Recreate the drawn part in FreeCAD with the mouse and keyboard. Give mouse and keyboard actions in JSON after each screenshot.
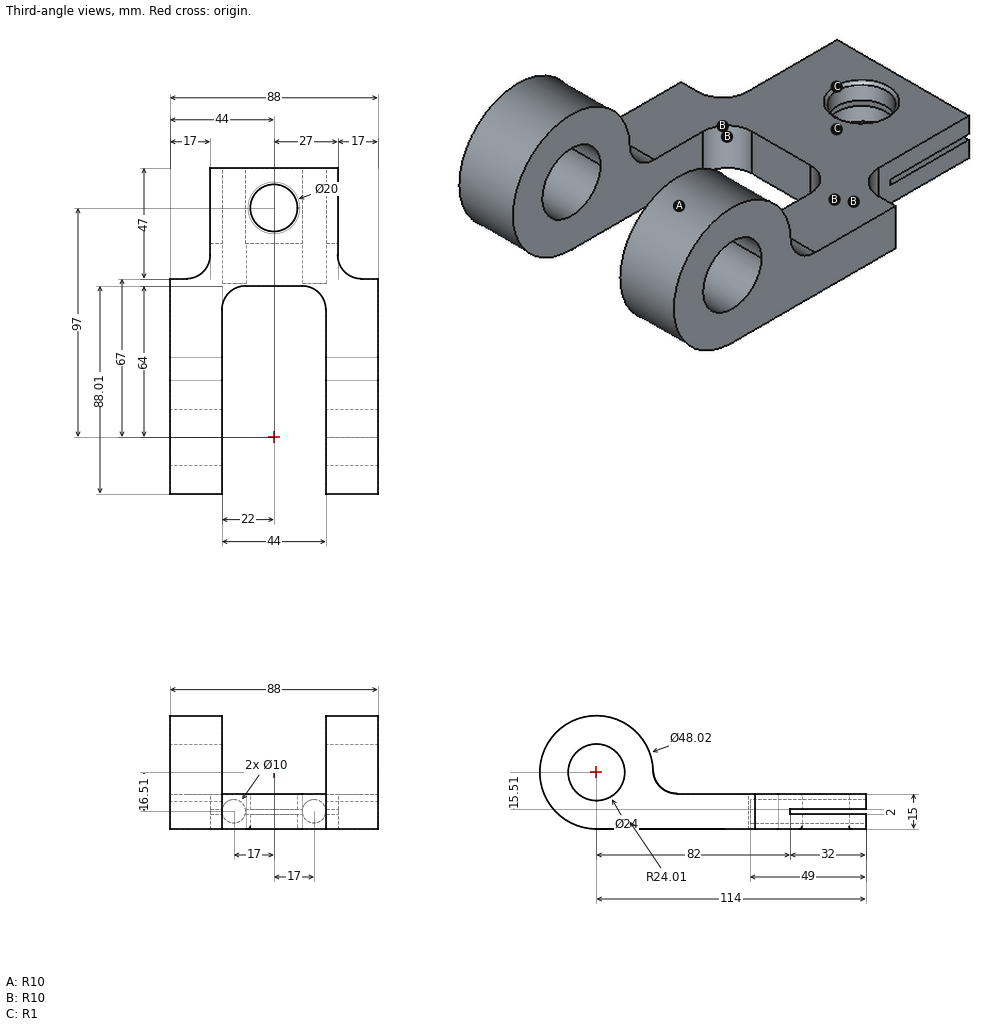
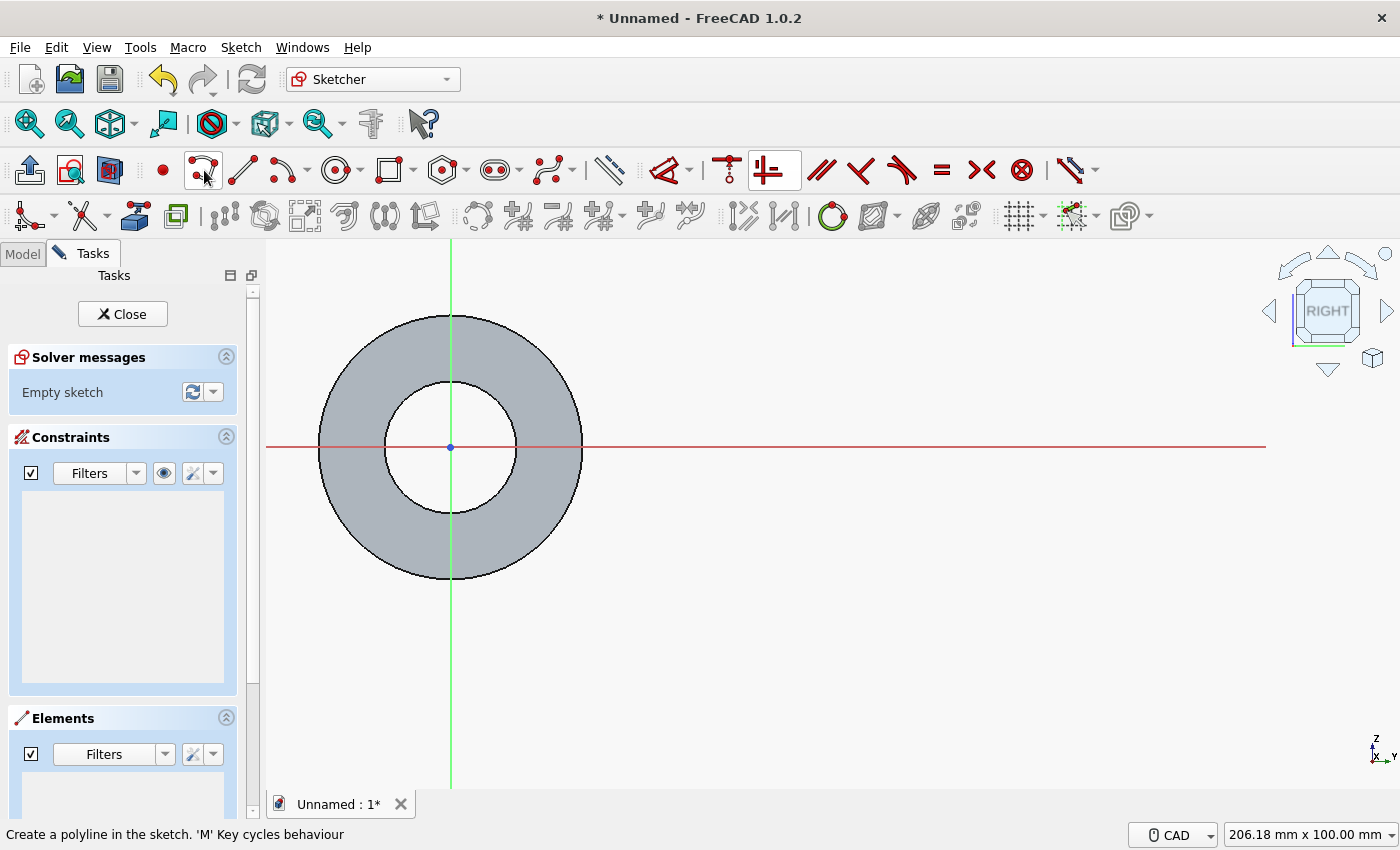
{"action": "left_click", "coordinate": [451, 580]}
{"action": "left_click", "coordinate": [1078, 580]}
{"action": "left_click", "coordinate": [1078, 497]}
{"action": "left_click", "coordinate": [573, 497]}
{"action": "right_click", "coordinate": [573, 497]}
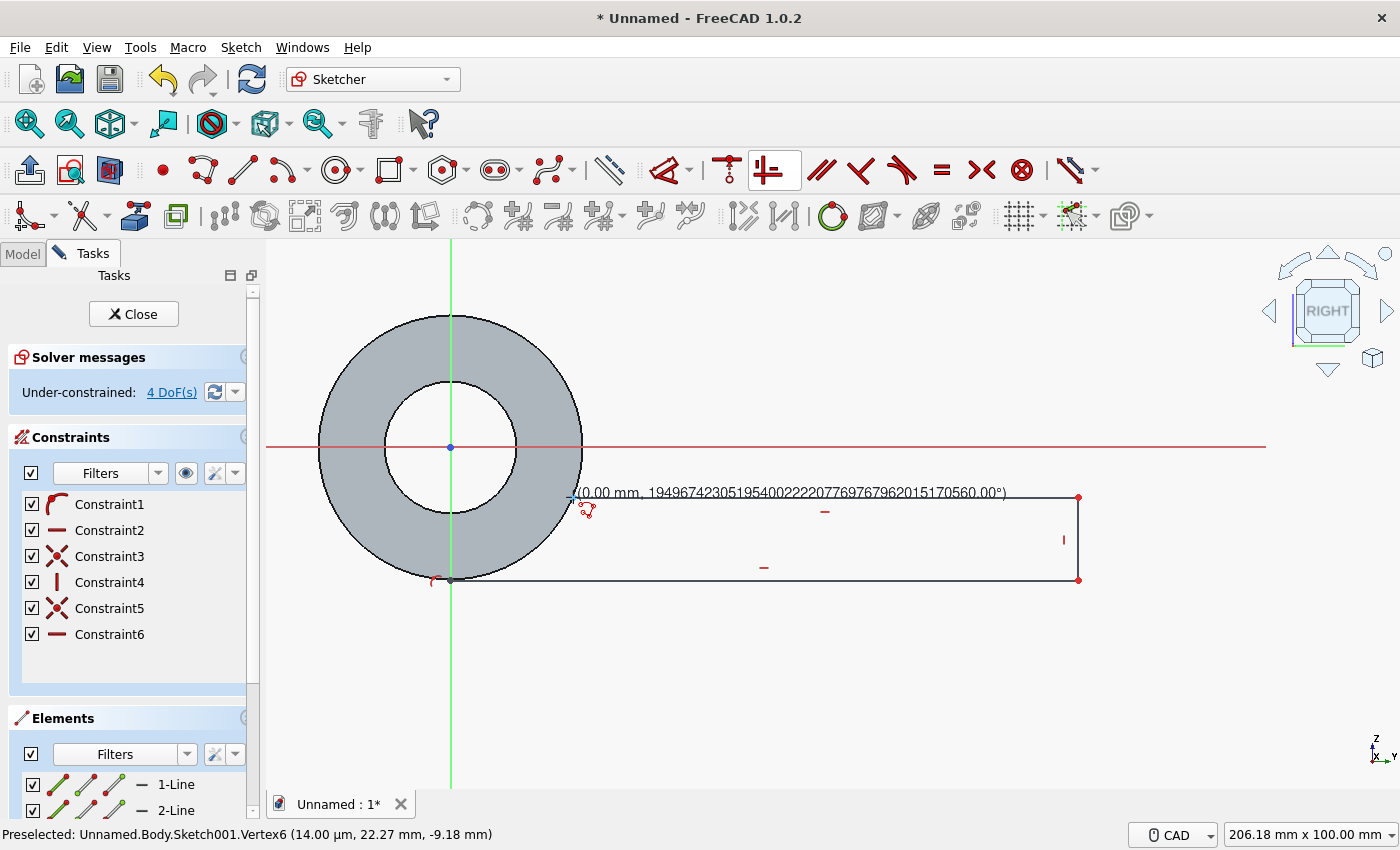
{"action": "left_click", "coordinate": [310, 170]}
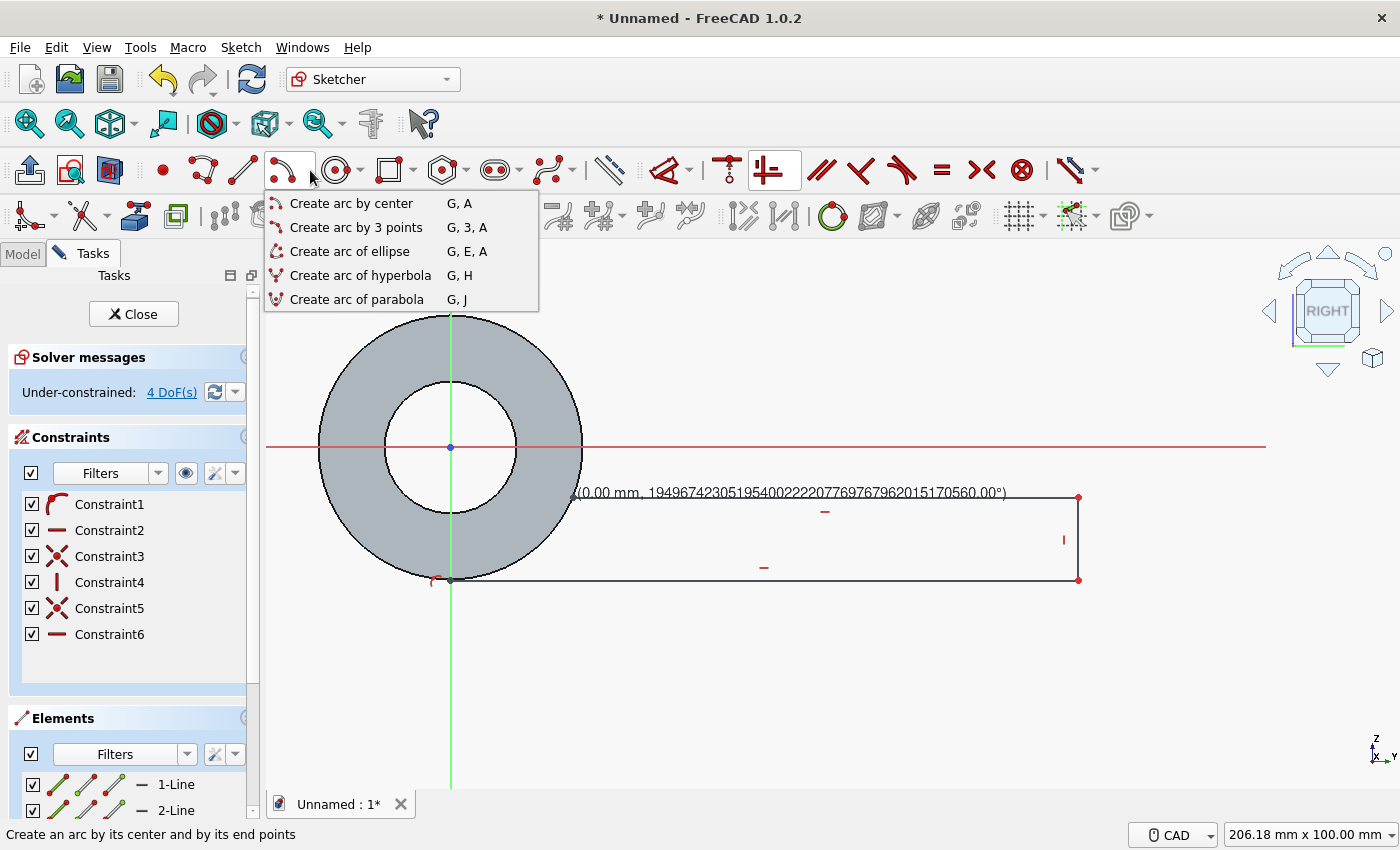
{"action": "left_click", "coordinate": [402, 227]}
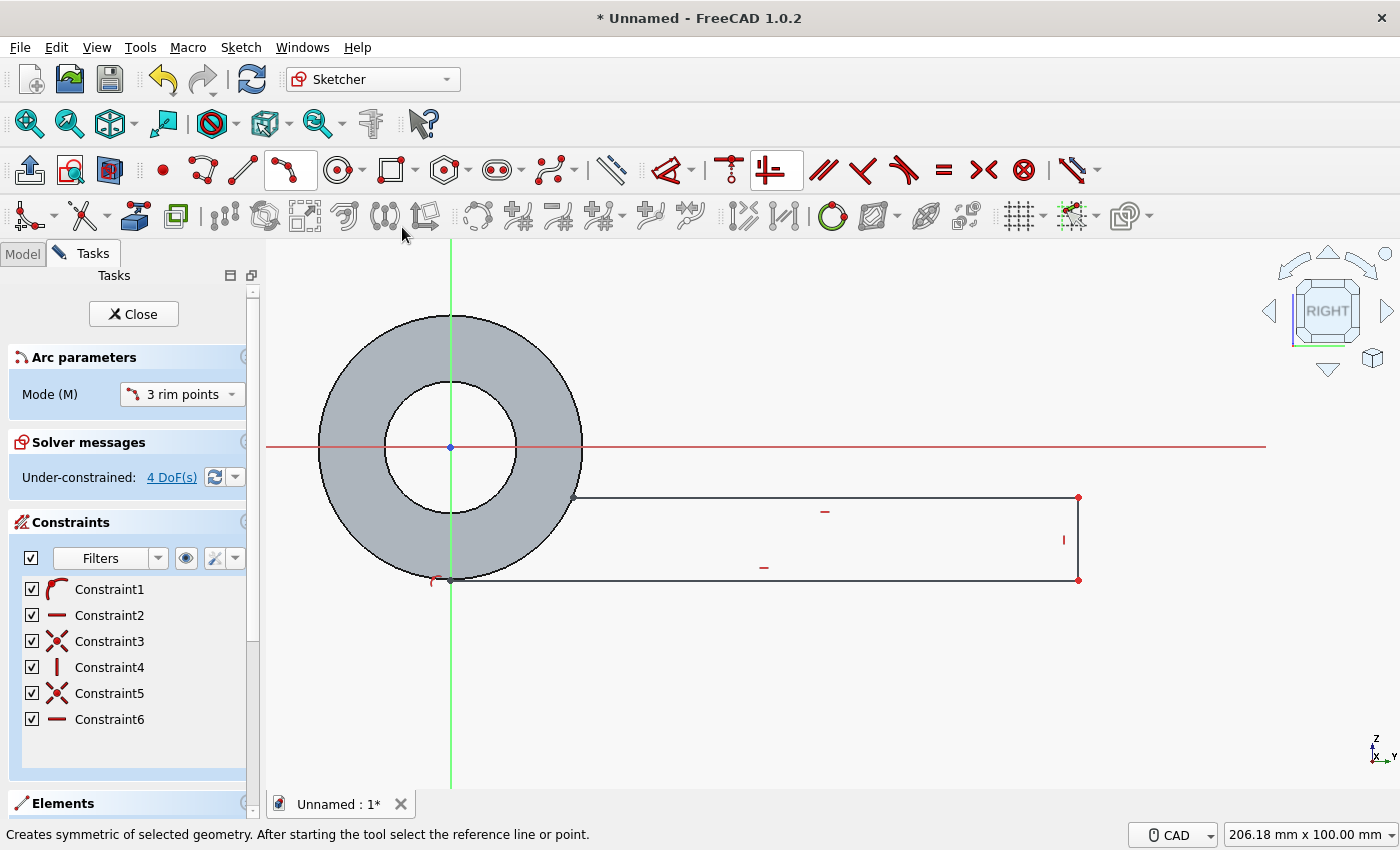
{"action": "left_click", "coordinate": [573, 498]}
{"action": "left_click", "coordinate": [451, 581]}
{"action": "left_click", "coordinate": [524, 557]}
{"action": "key", "text": "Escape"}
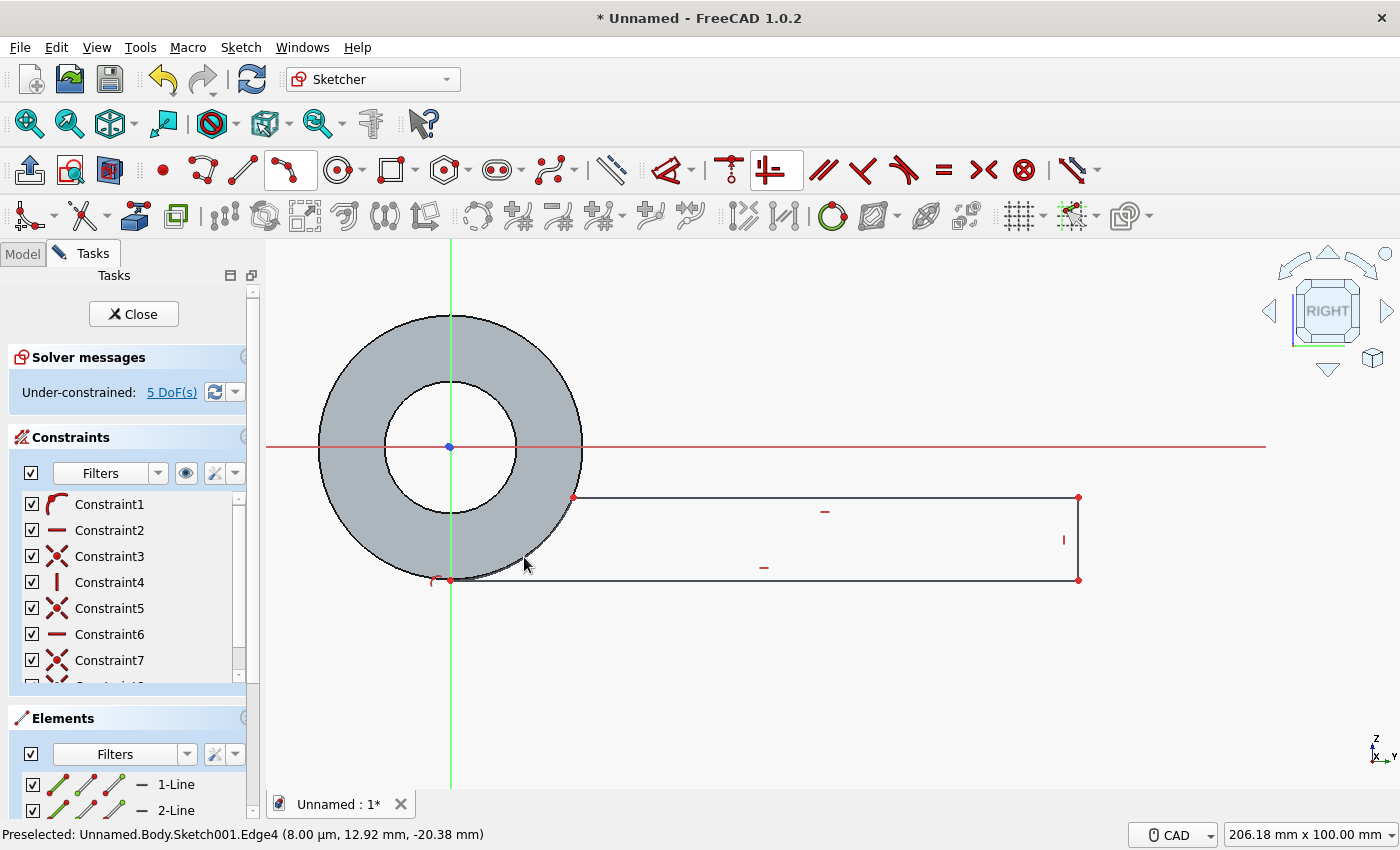
{"action": "left_click", "coordinate": [639, 581]}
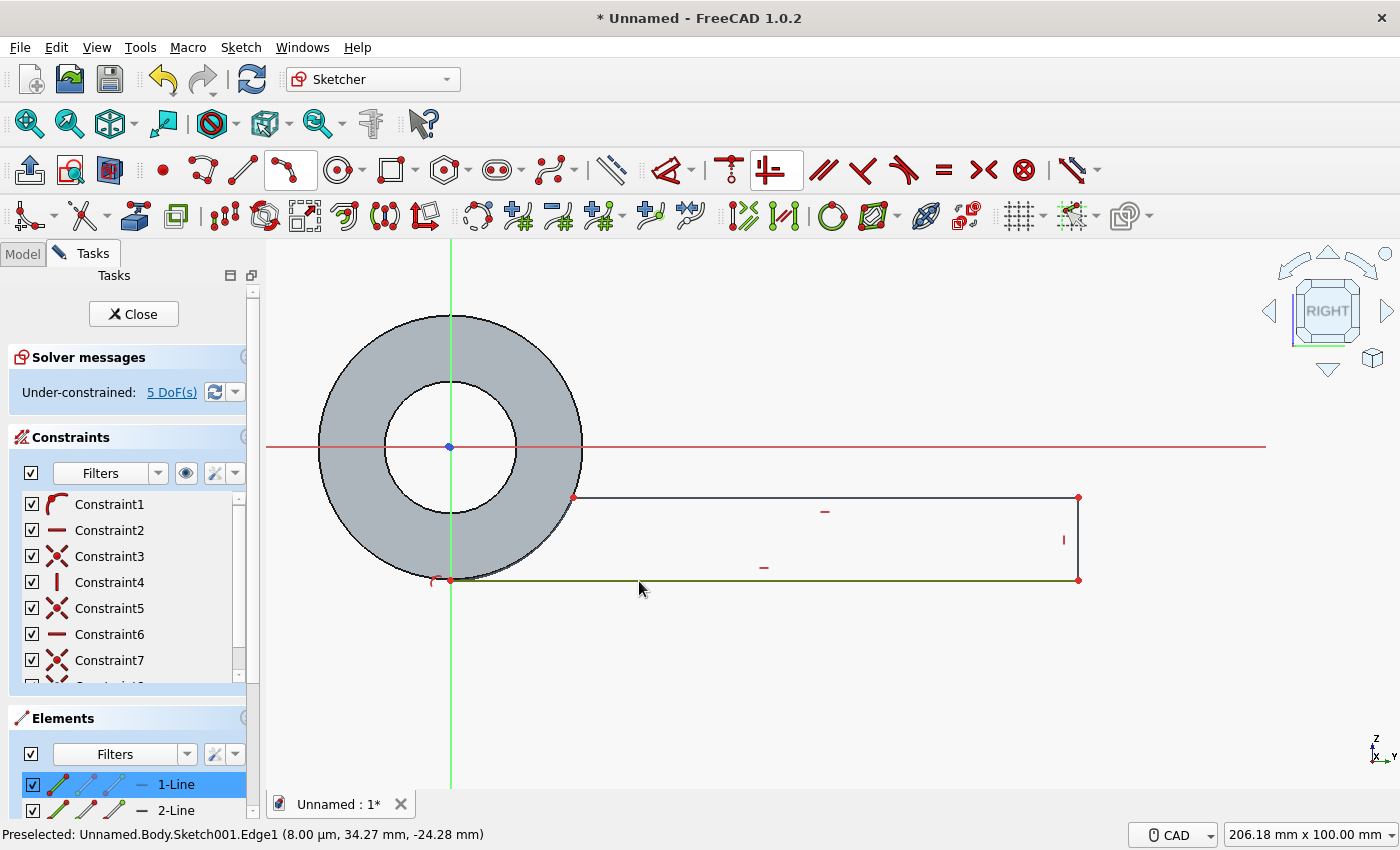
{"action": "left_click", "coordinate": [548, 537]}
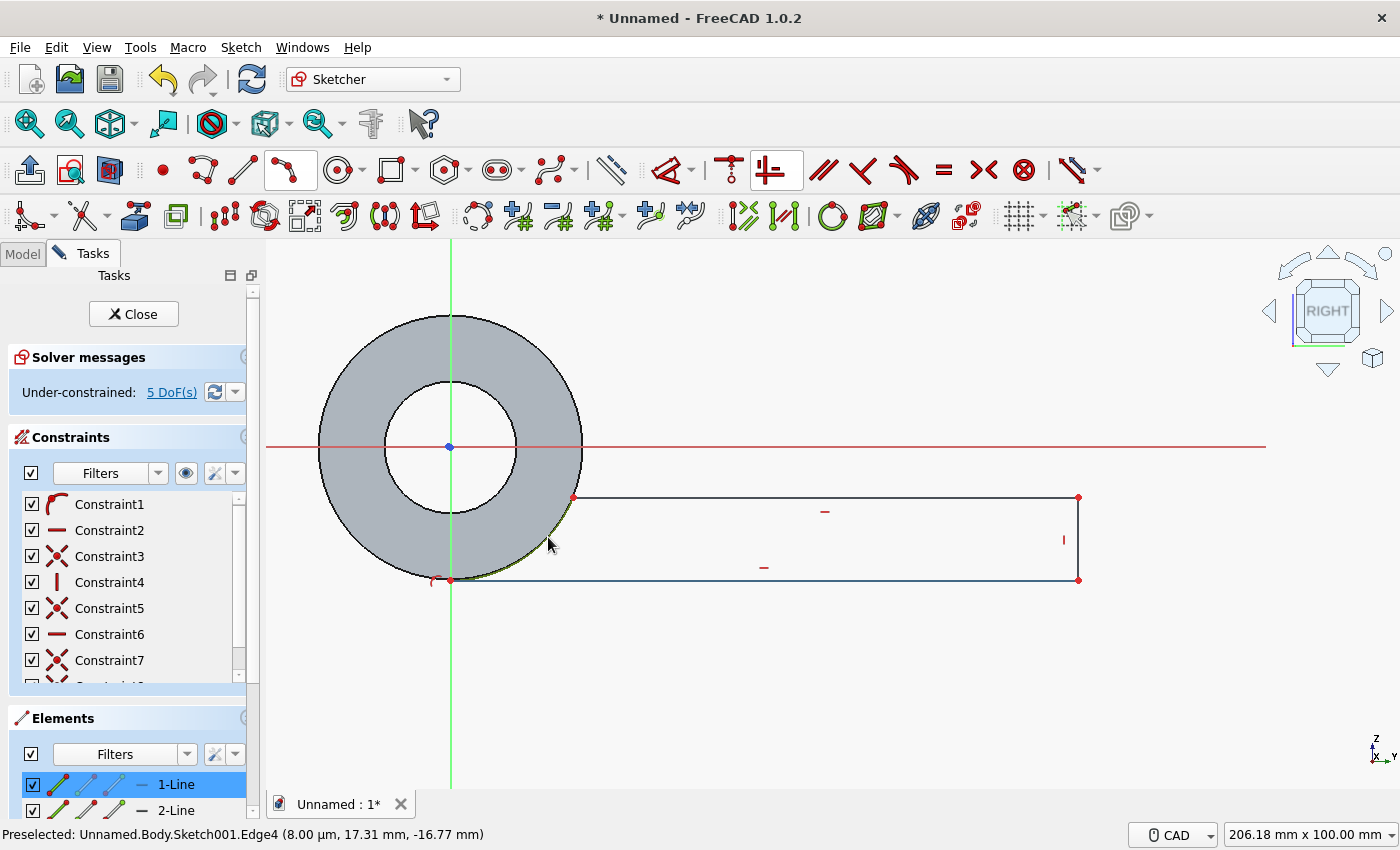
{"action": "left_click", "coordinate": [904, 170]}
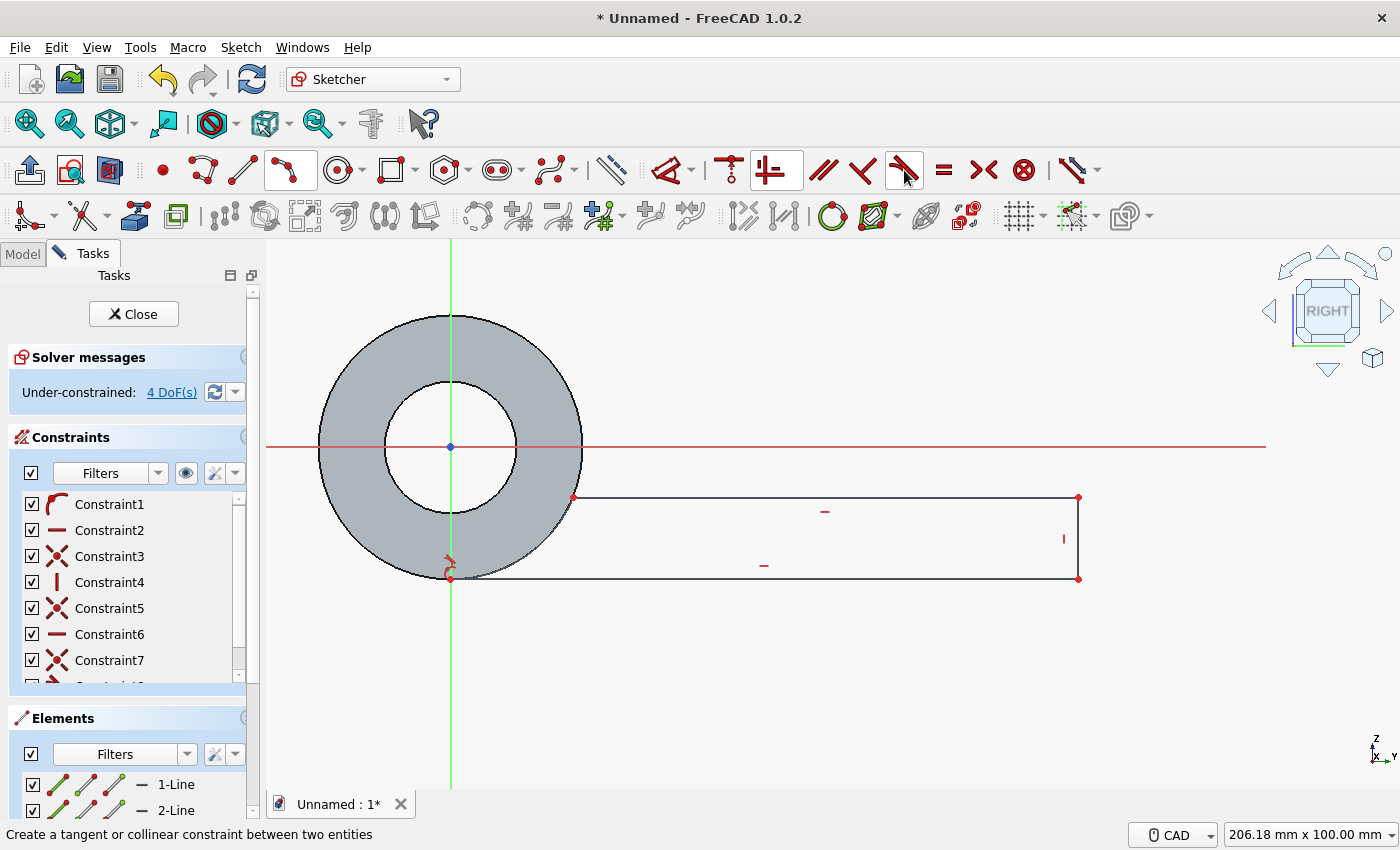
{"action": "left_click", "coordinate": [451, 447]}